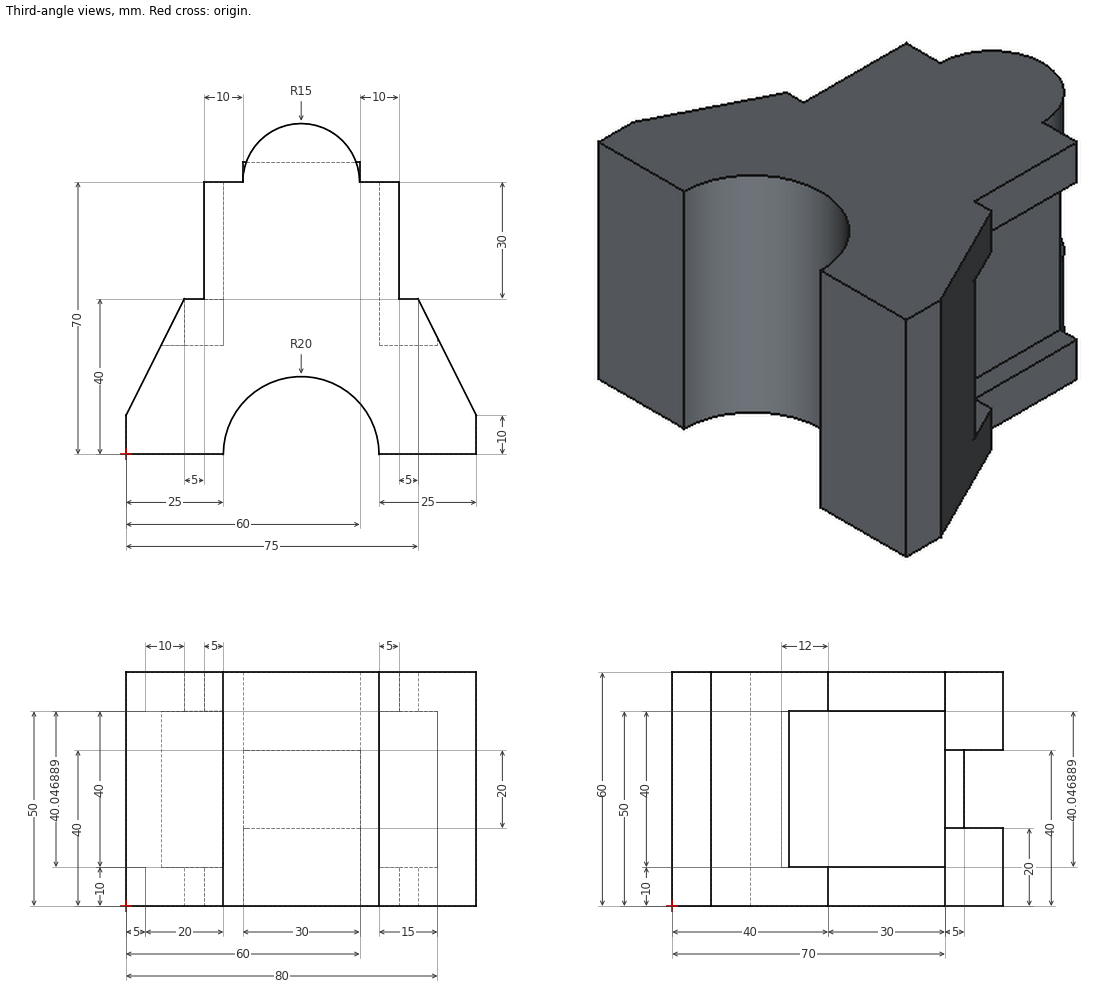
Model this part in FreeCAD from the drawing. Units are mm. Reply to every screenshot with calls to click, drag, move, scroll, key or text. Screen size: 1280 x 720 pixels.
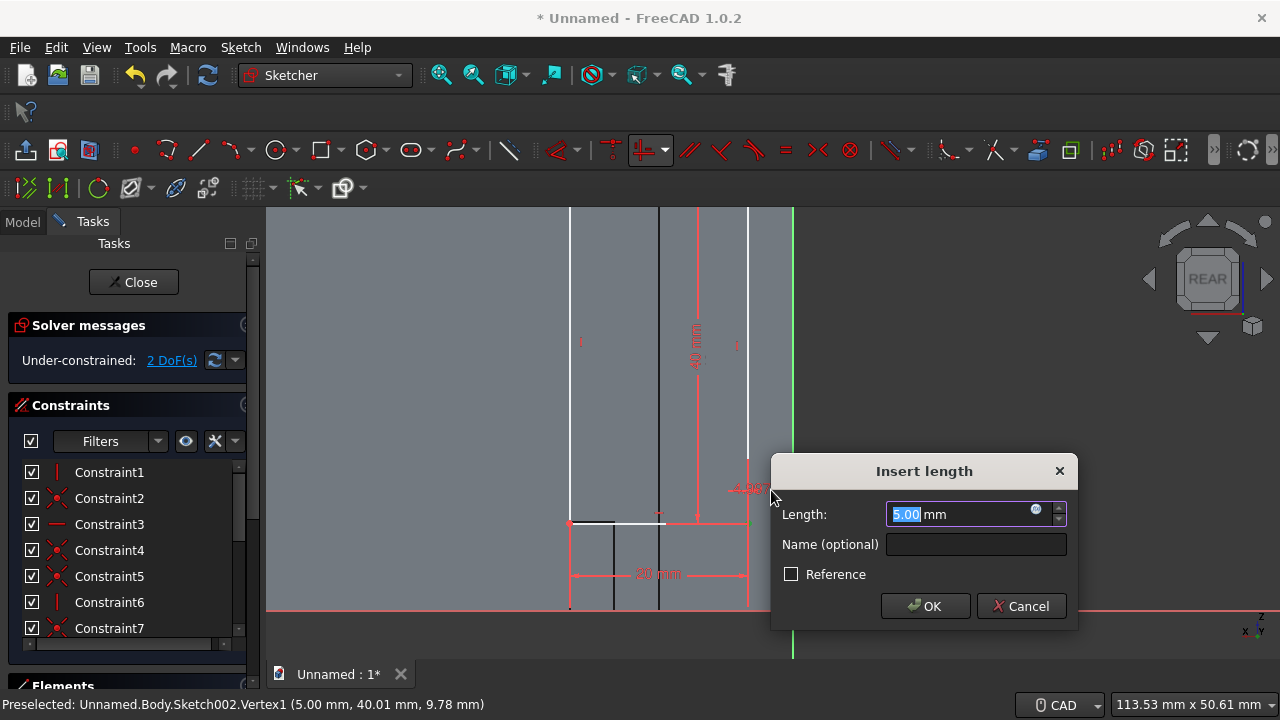
text(5)
key(Return)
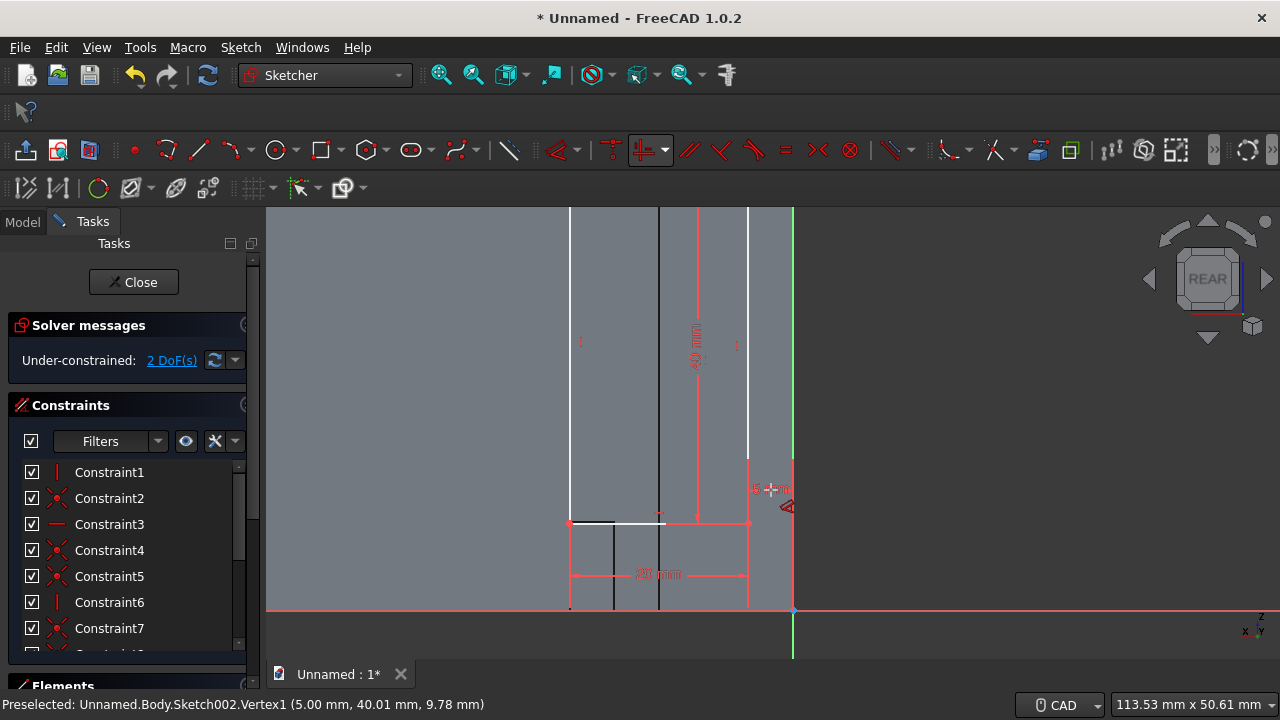
click(748, 524)
click(827, 567)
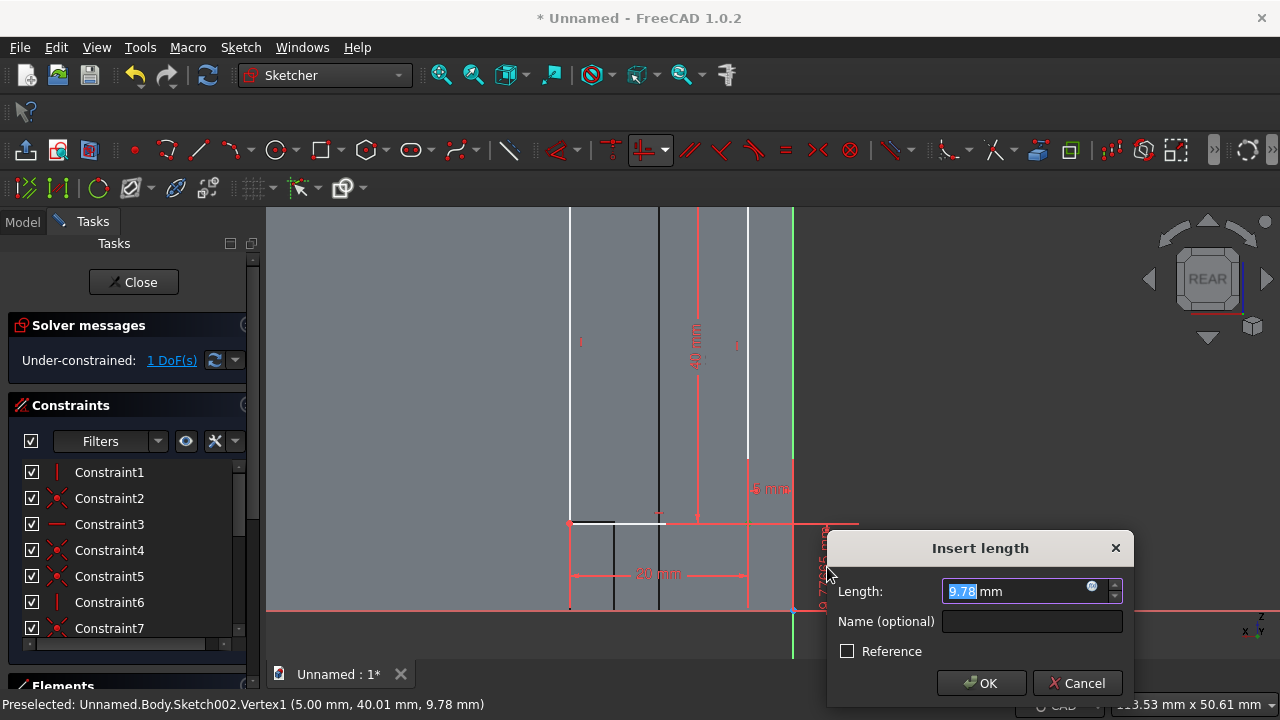
text(10)
key(Return)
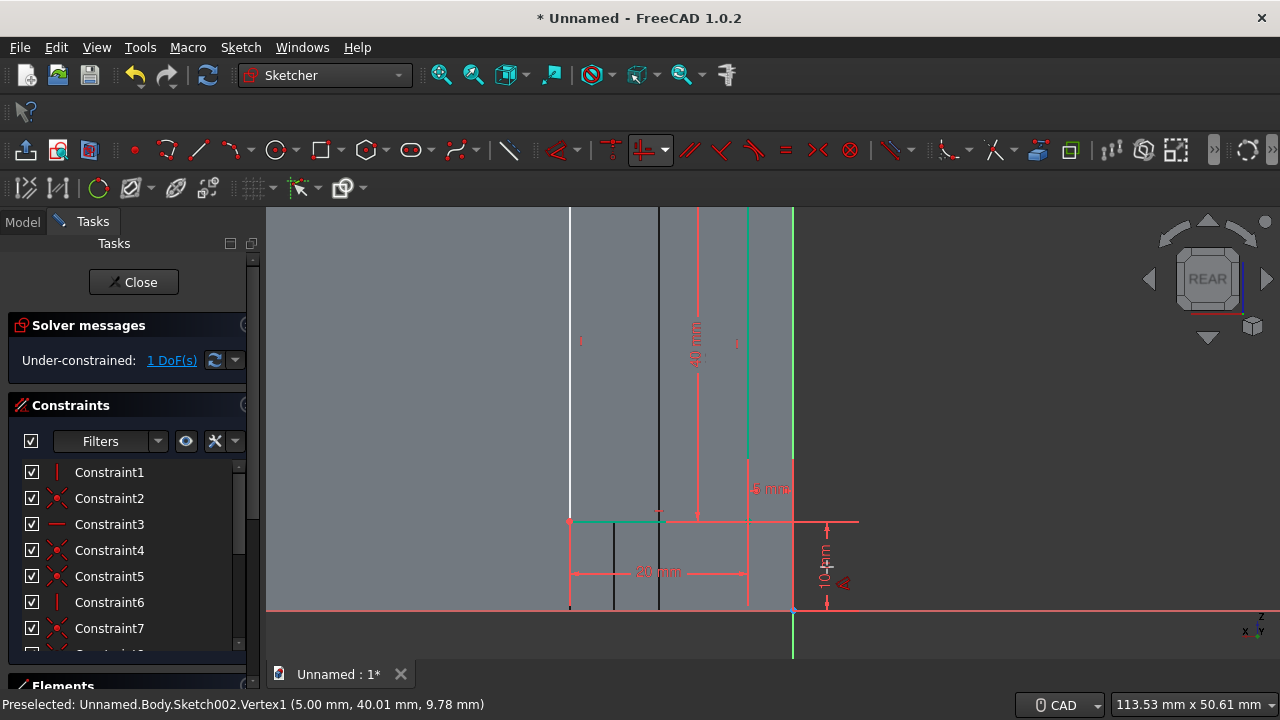
click(570, 268)
click(536, 378)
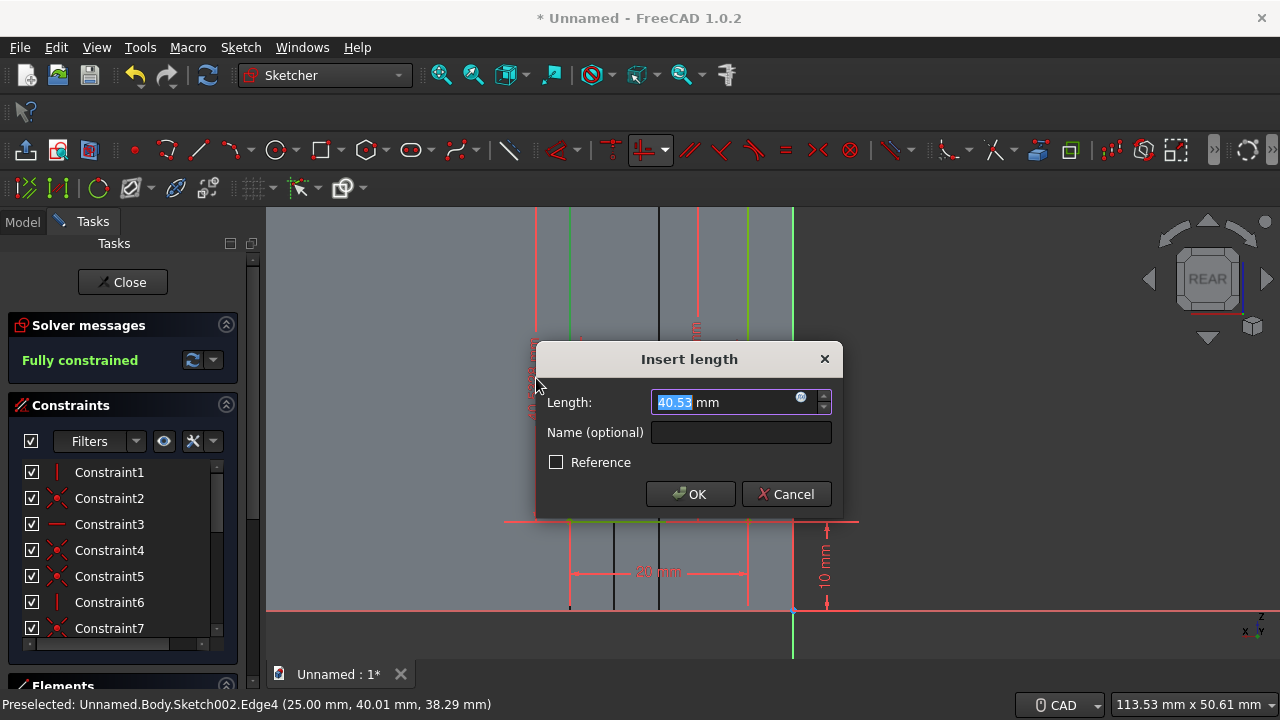
text(40.046889)
key(Return)
key(Escape)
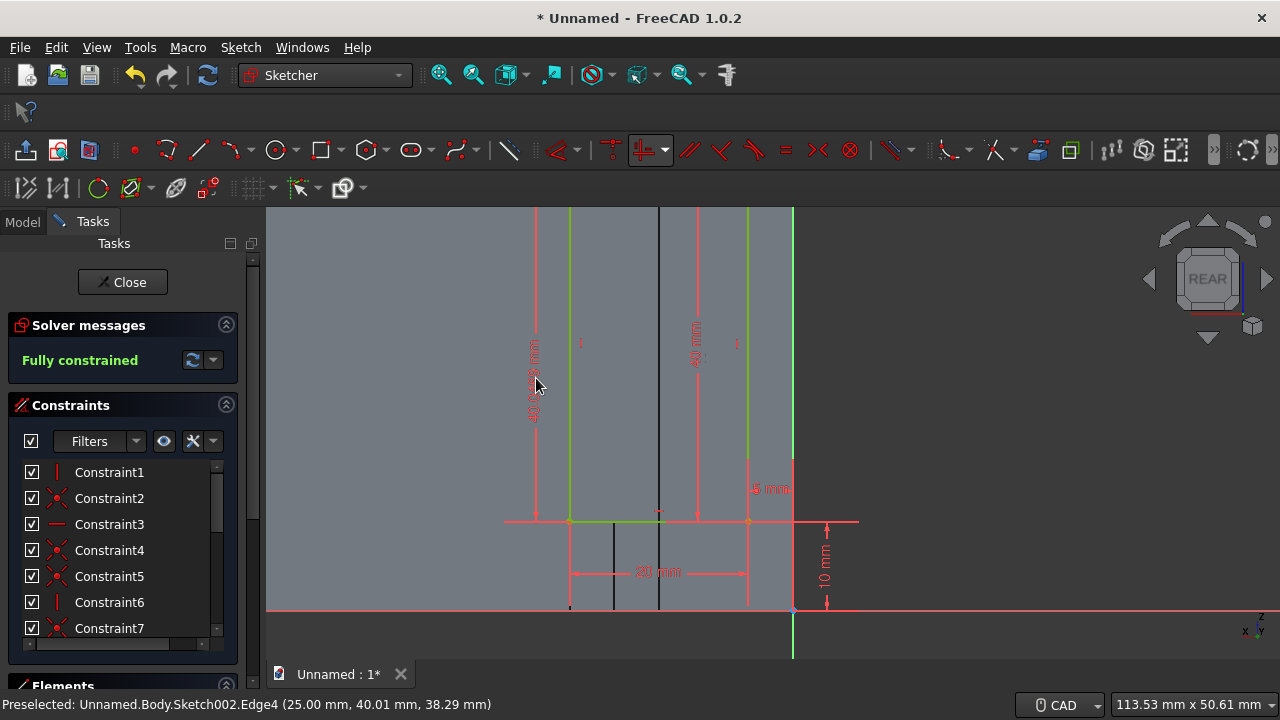
click(123, 282)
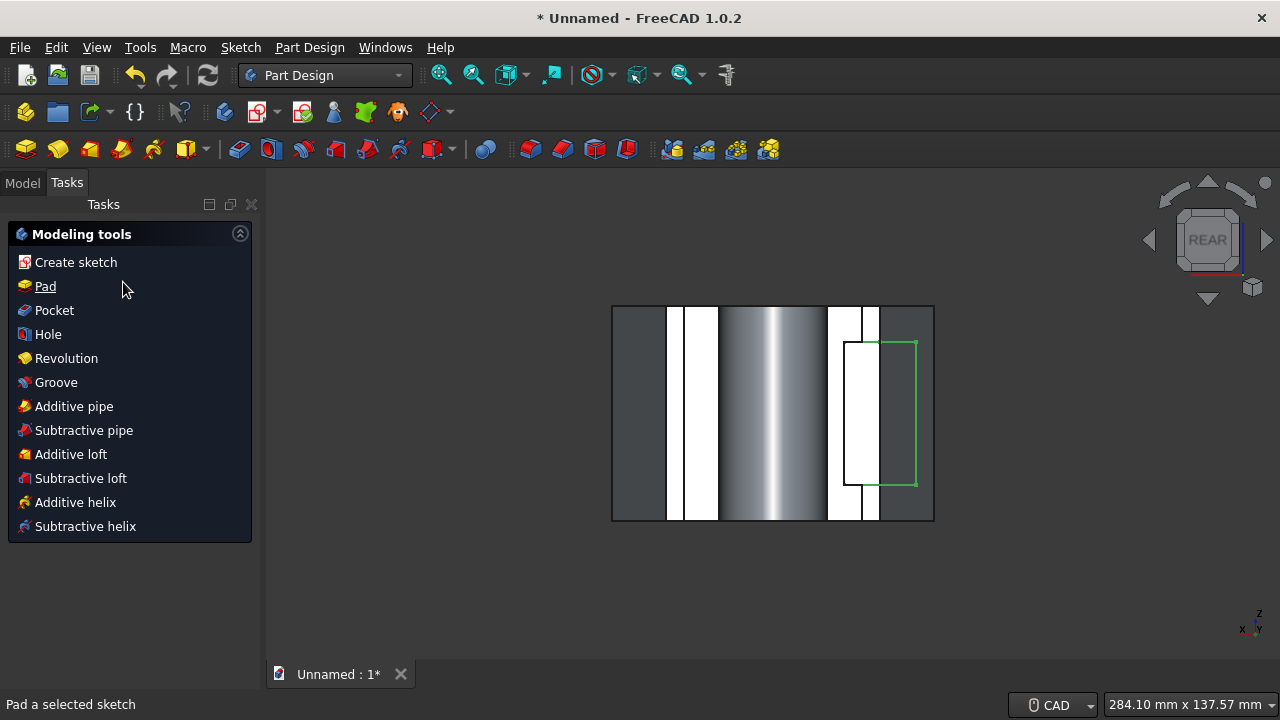
click(240, 150)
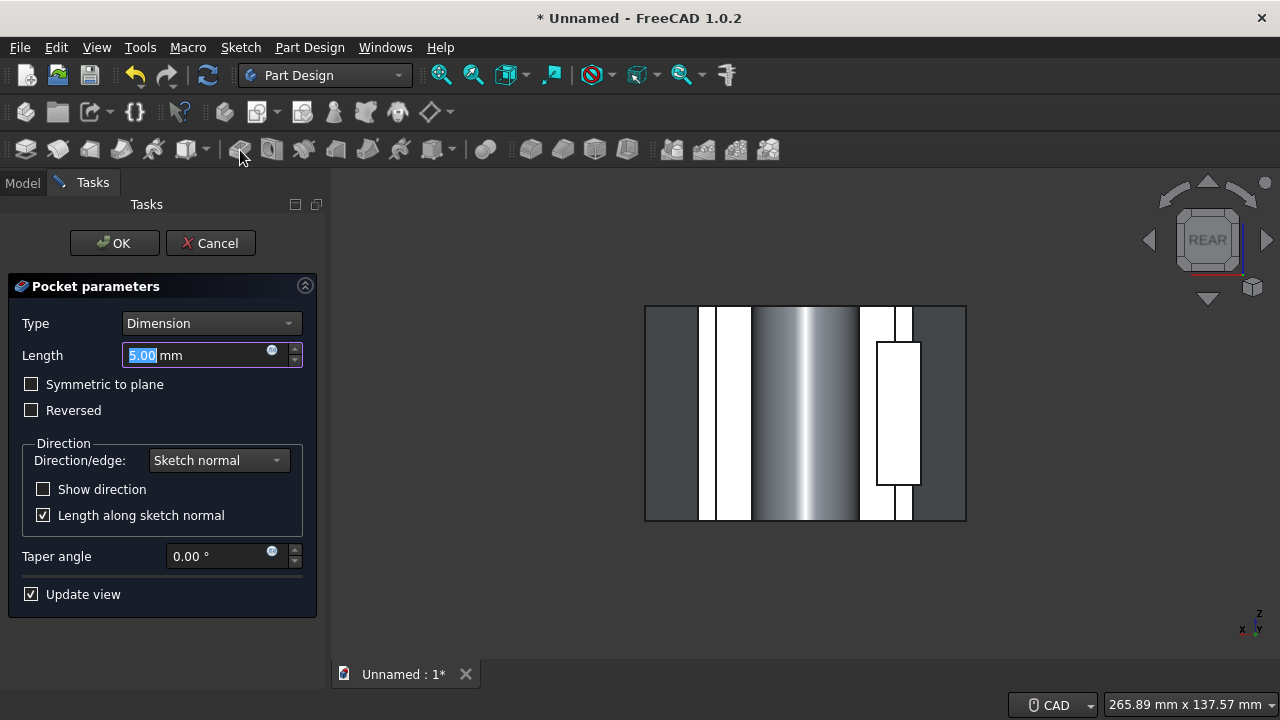
text(12)
key(Tab)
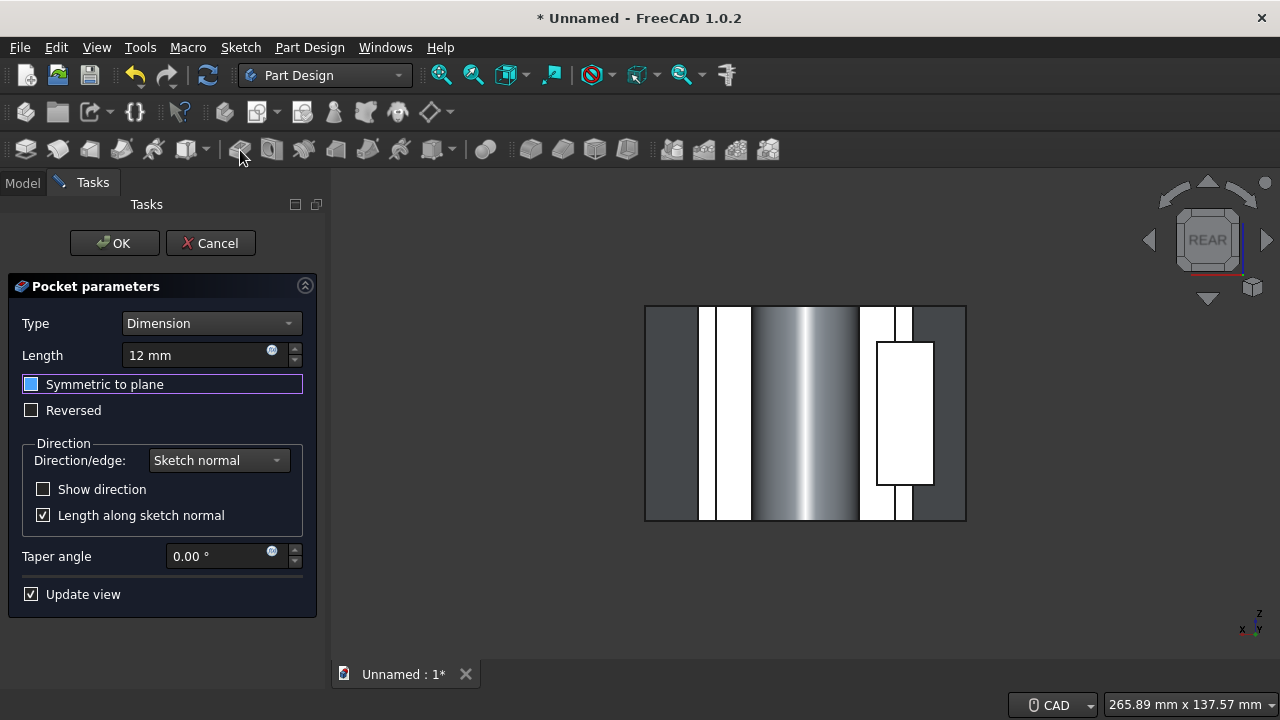
click(115, 243)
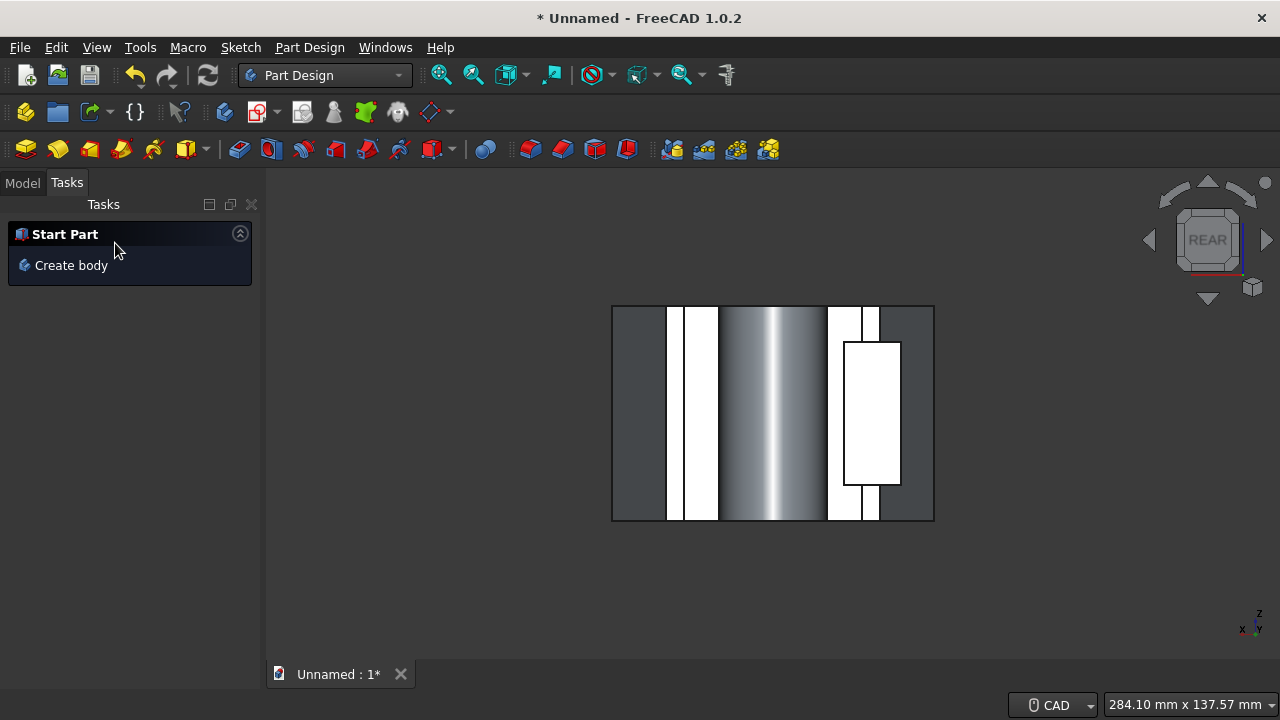
key(v)
key(f)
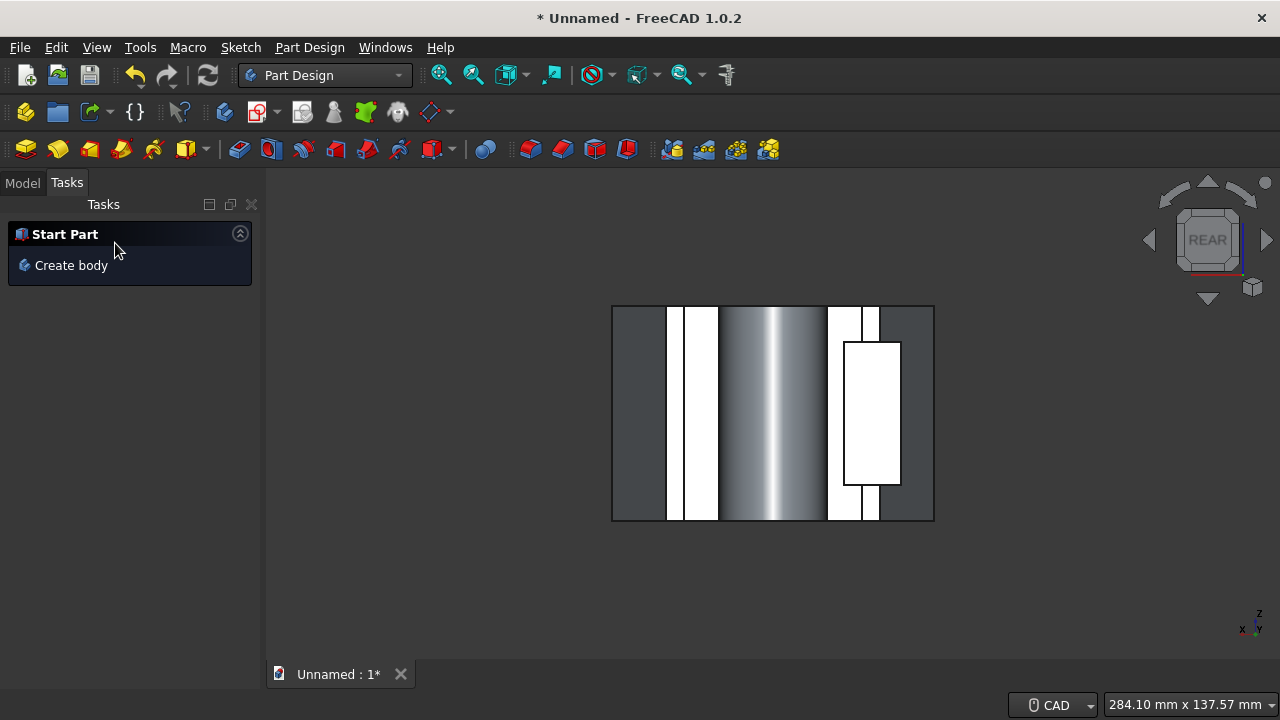
key(0)